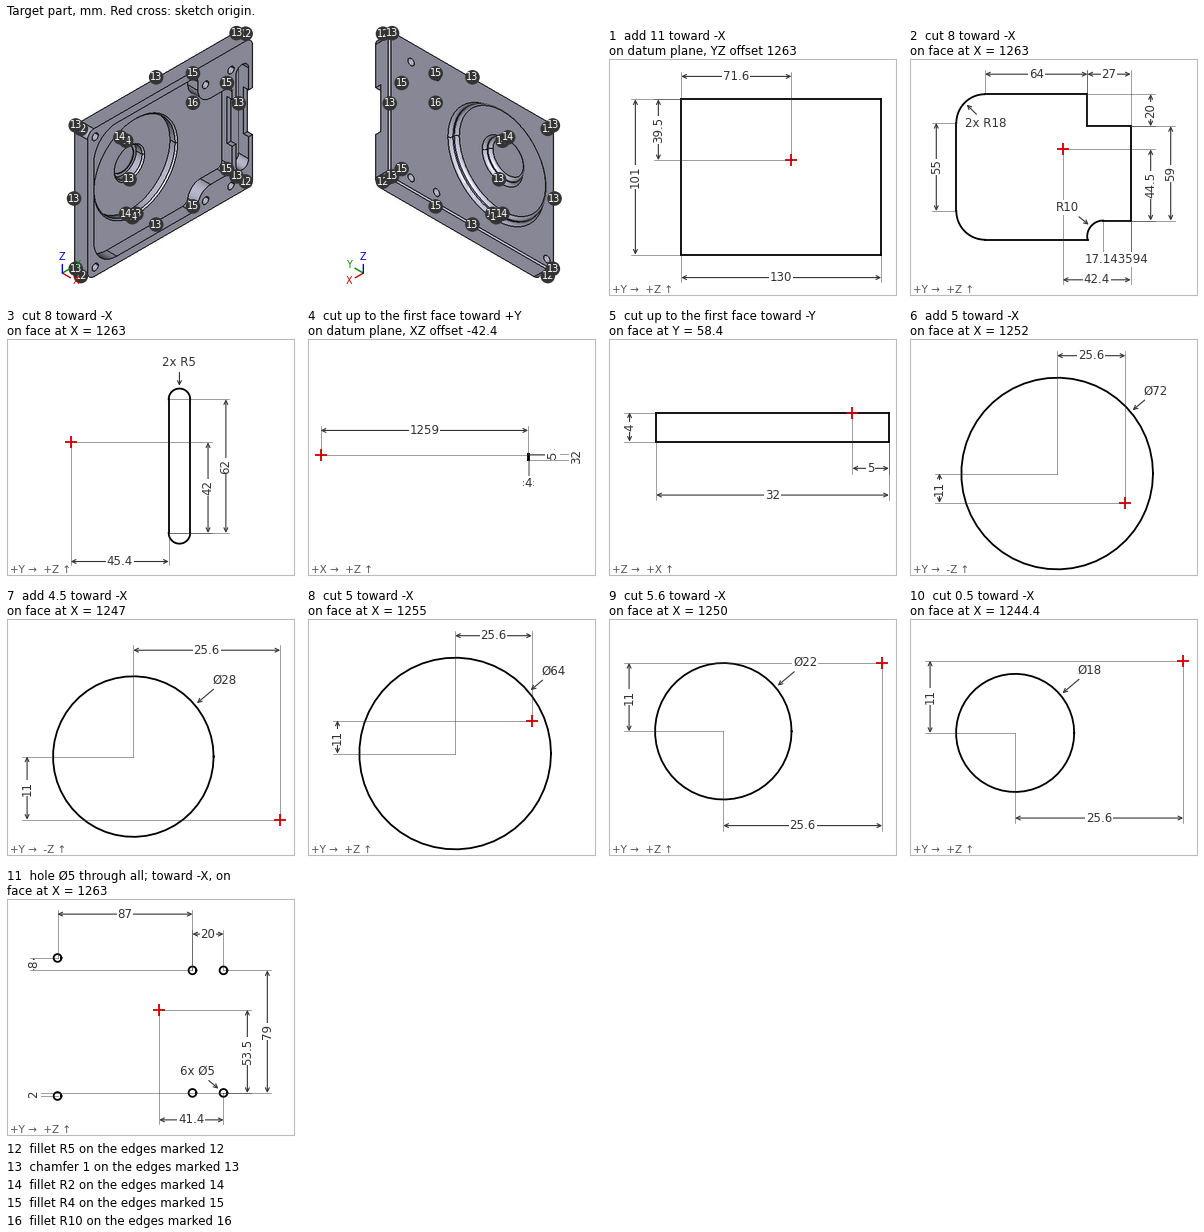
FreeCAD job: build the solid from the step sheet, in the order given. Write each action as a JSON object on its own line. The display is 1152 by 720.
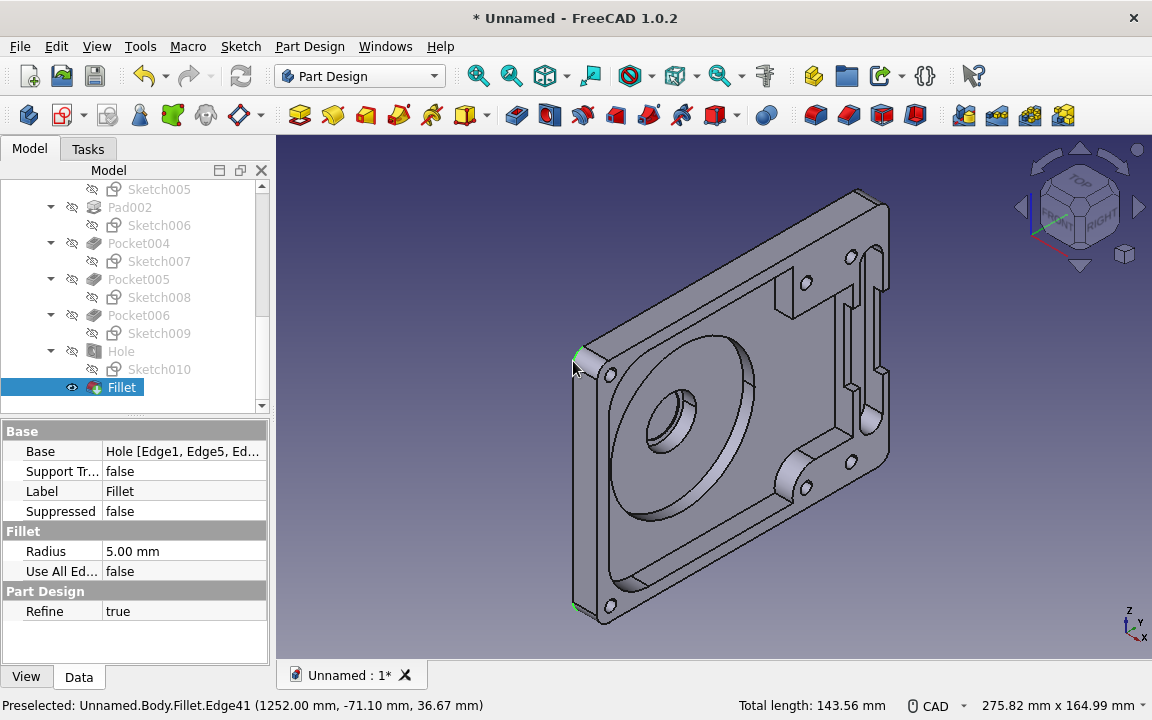
{"action": "left_click", "coordinate": [660, 519], "text": "ctrl"}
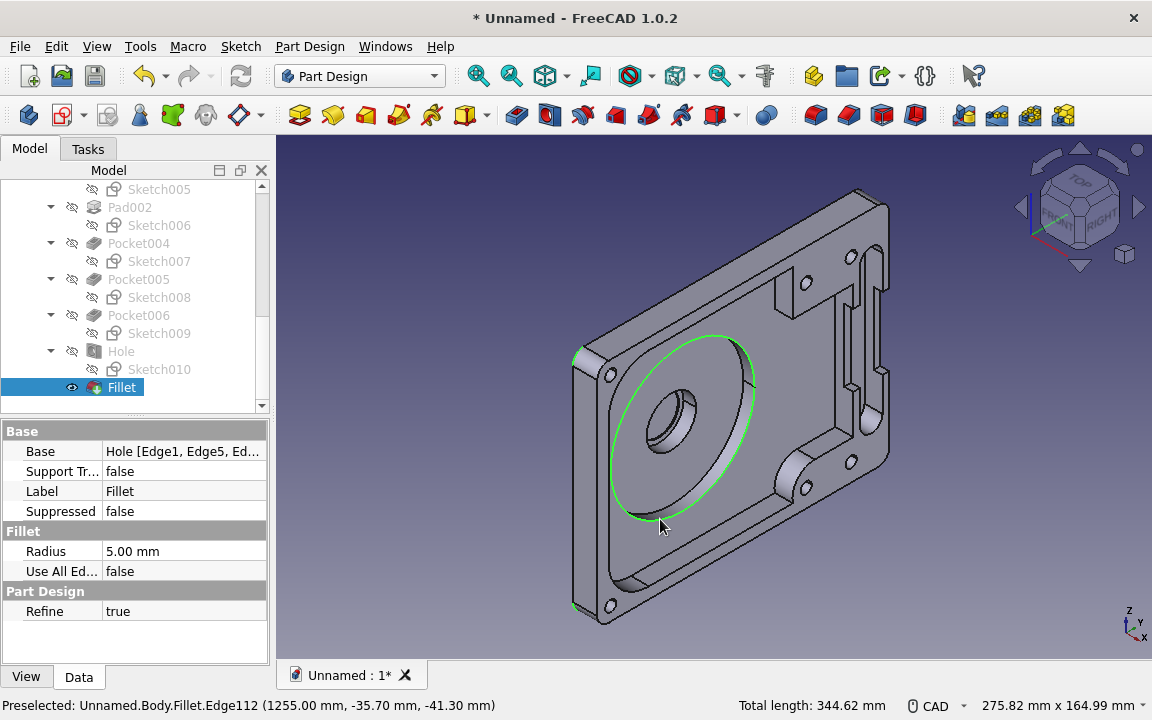
{"action": "left_click", "coordinate": [664, 452], "text": "ctrl"}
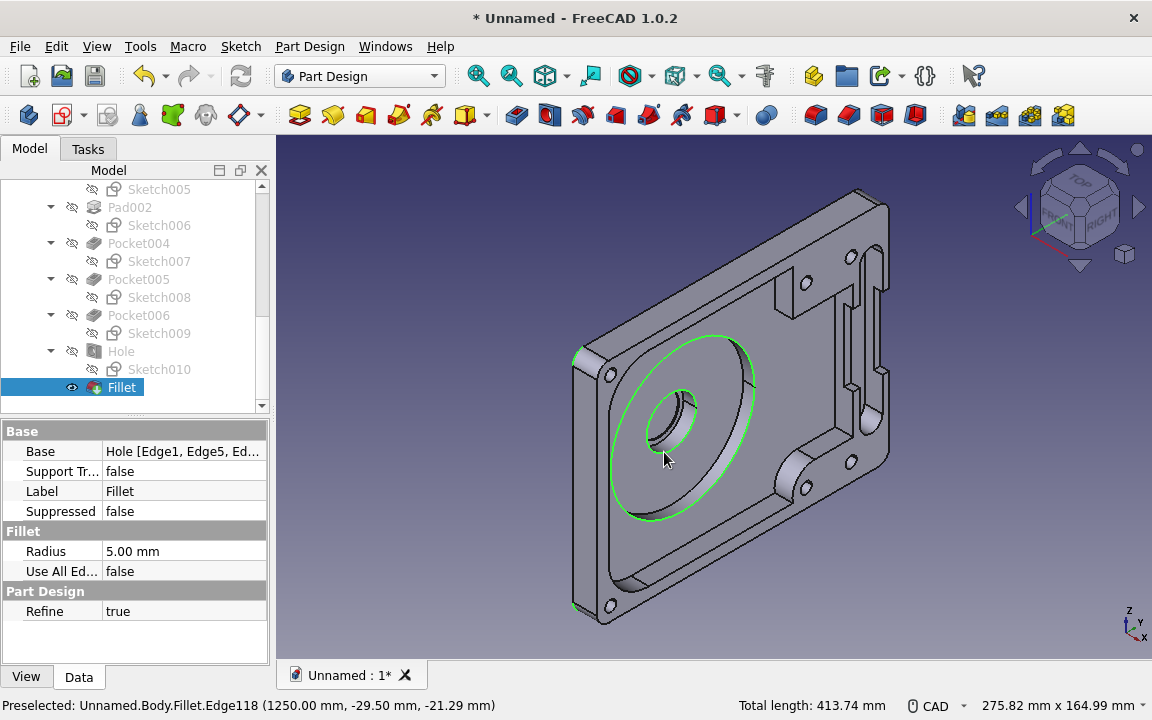
{"action": "key", "text": "2"}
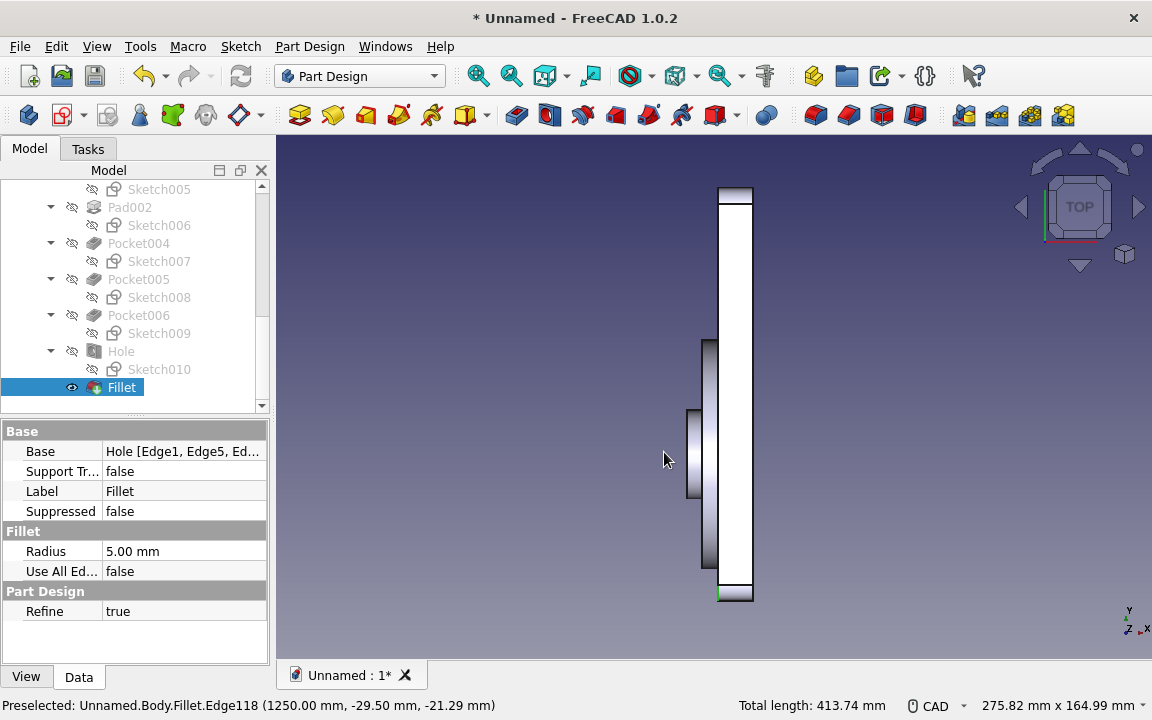
{"action": "left_click", "coordinate": [718, 393], "text": "ctrl"}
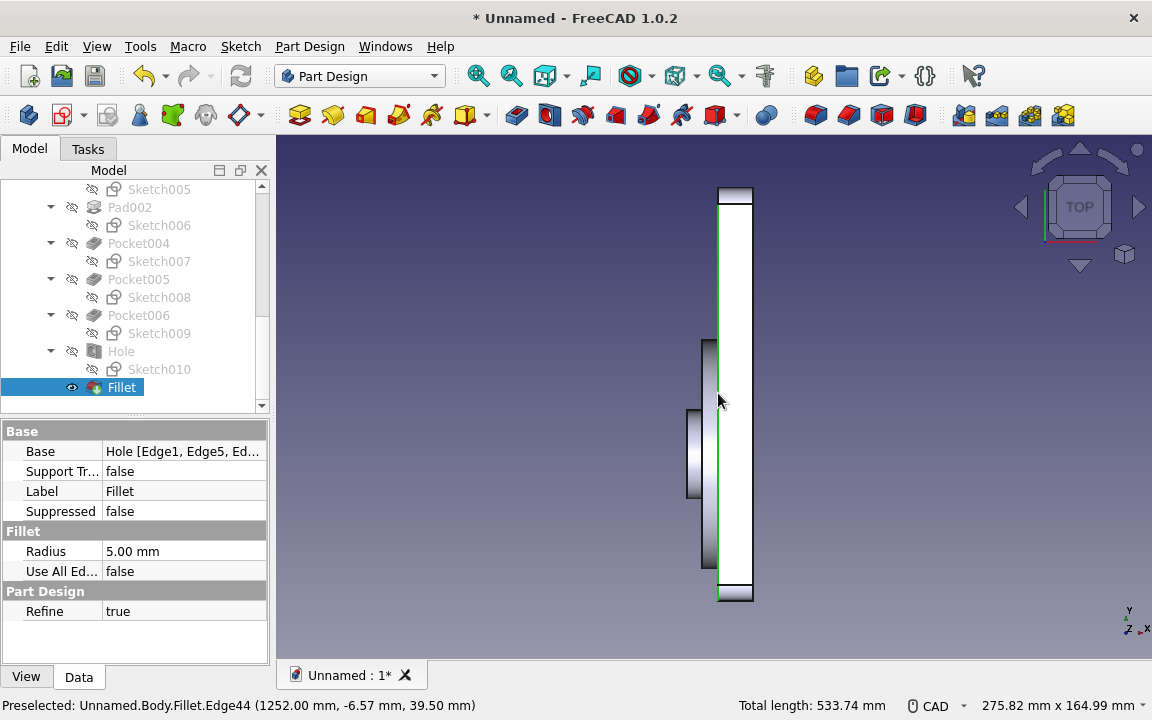
{"action": "left_click", "coordinate": [718, 191], "text": "ctrl"}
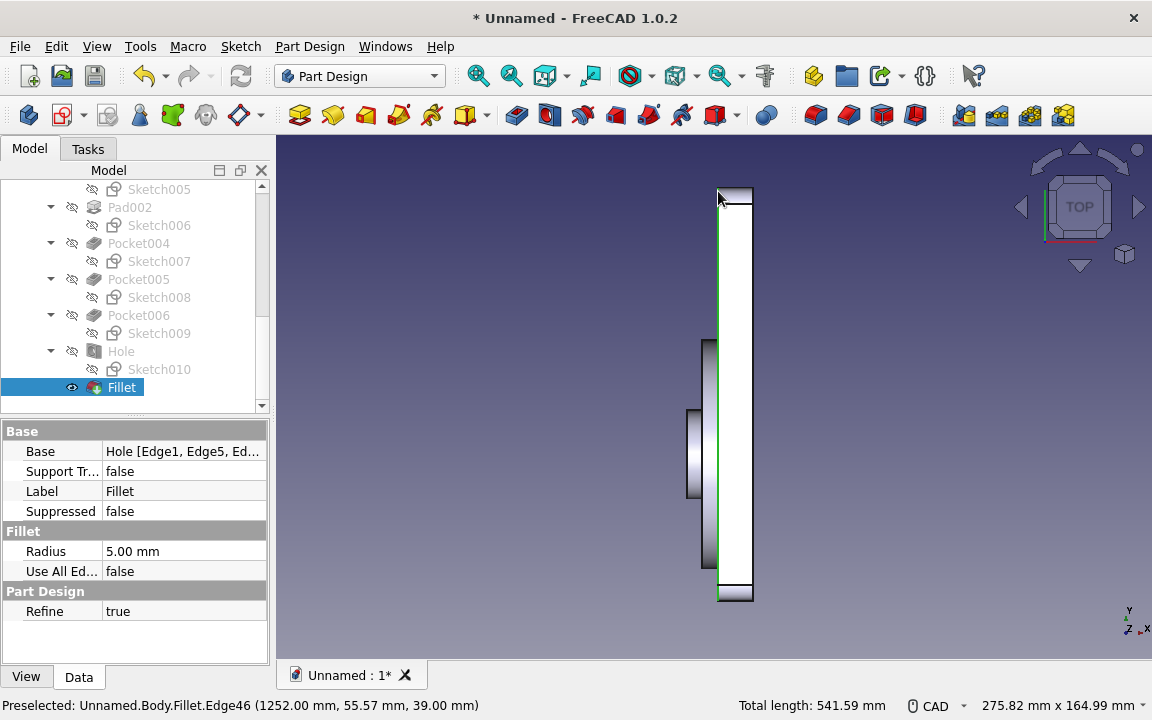
{"action": "key", "text": "1"}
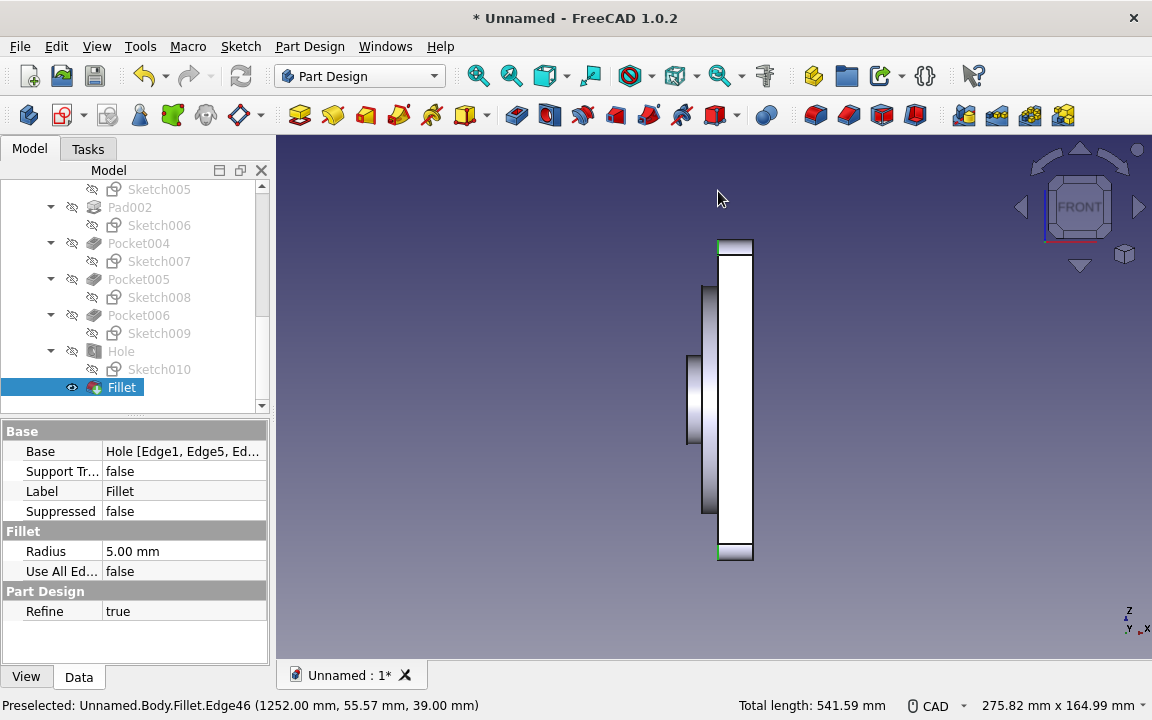
{"action": "left_click", "coordinate": [718, 399], "text": "ctrl"}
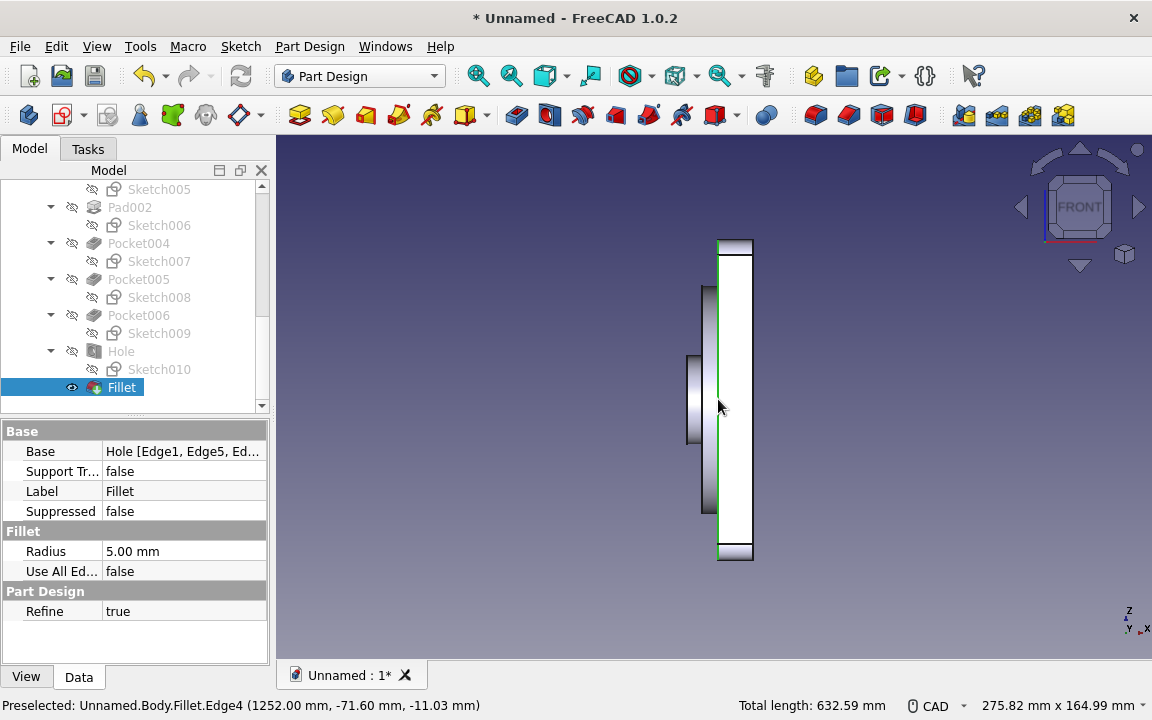
{"action": "key", "text": "3"}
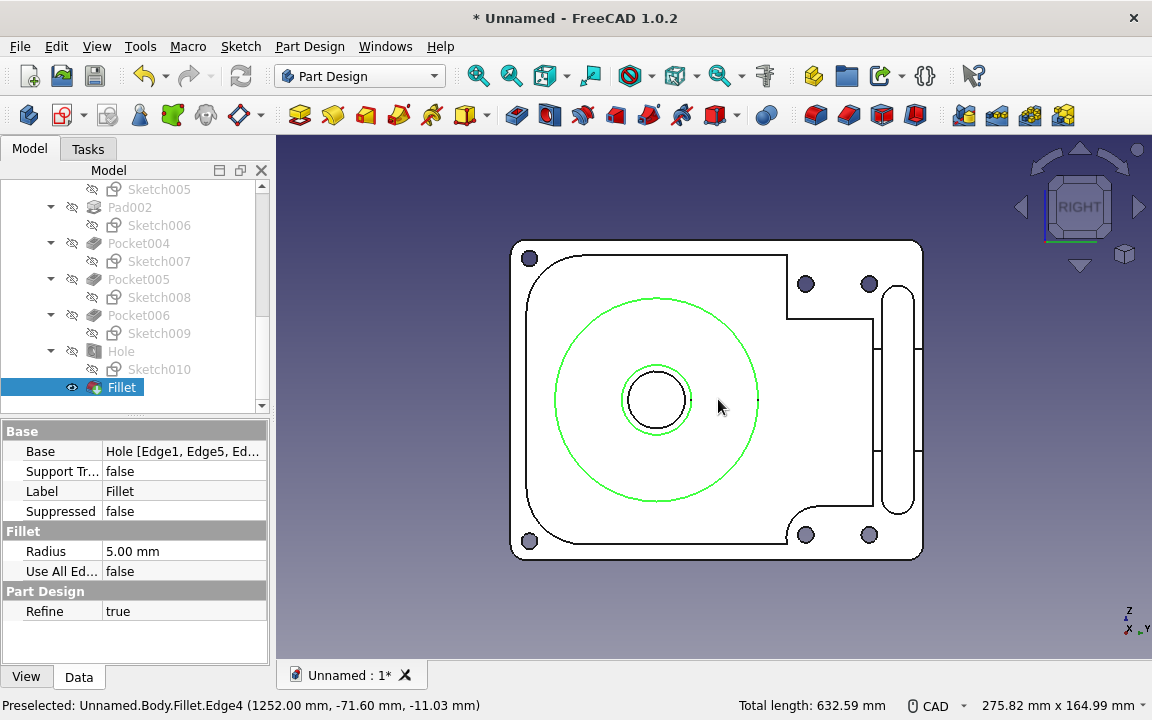
{"action": "key", "text": "5"}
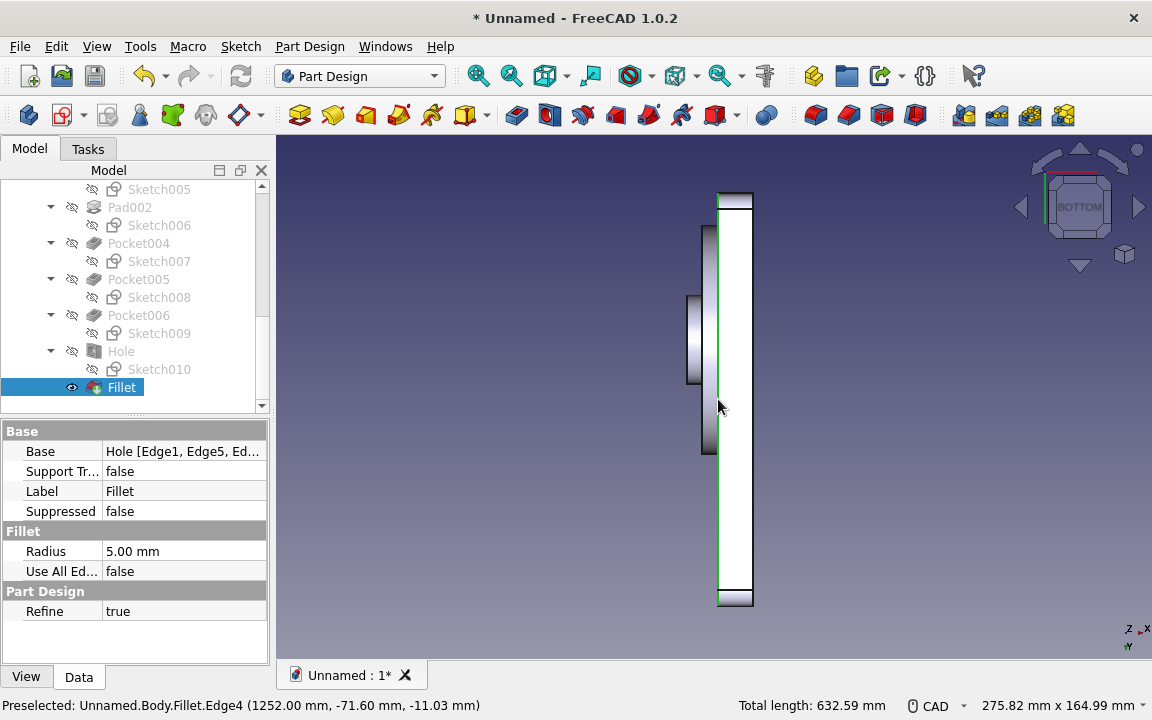
{"action": "key", "text": "4"}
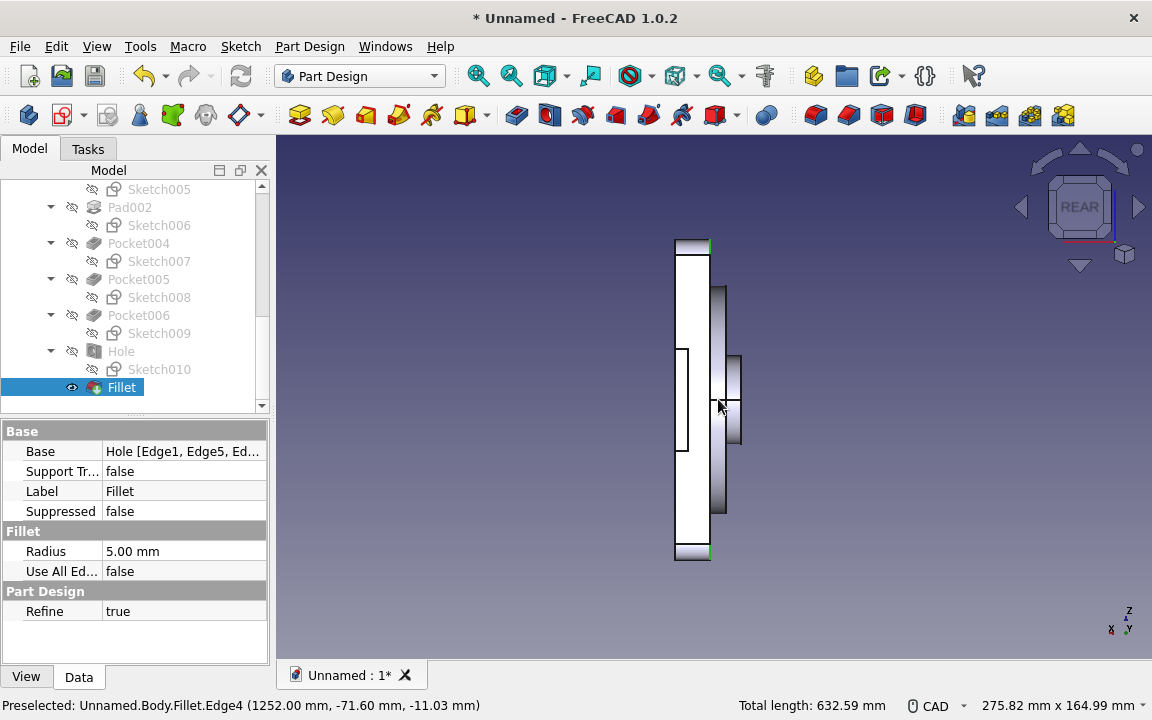
{"action": "left_click", "coordinate": [710, 399], "text": "ctrl"}